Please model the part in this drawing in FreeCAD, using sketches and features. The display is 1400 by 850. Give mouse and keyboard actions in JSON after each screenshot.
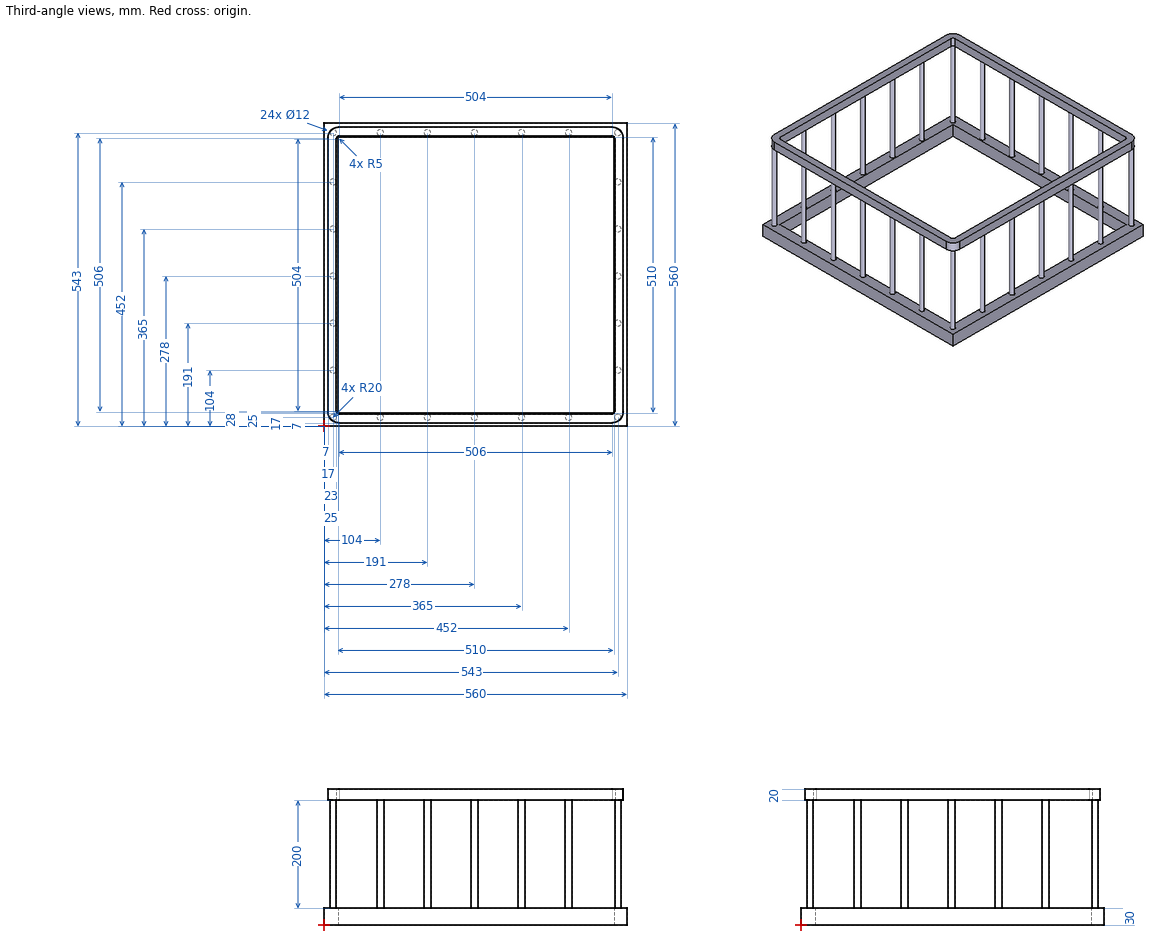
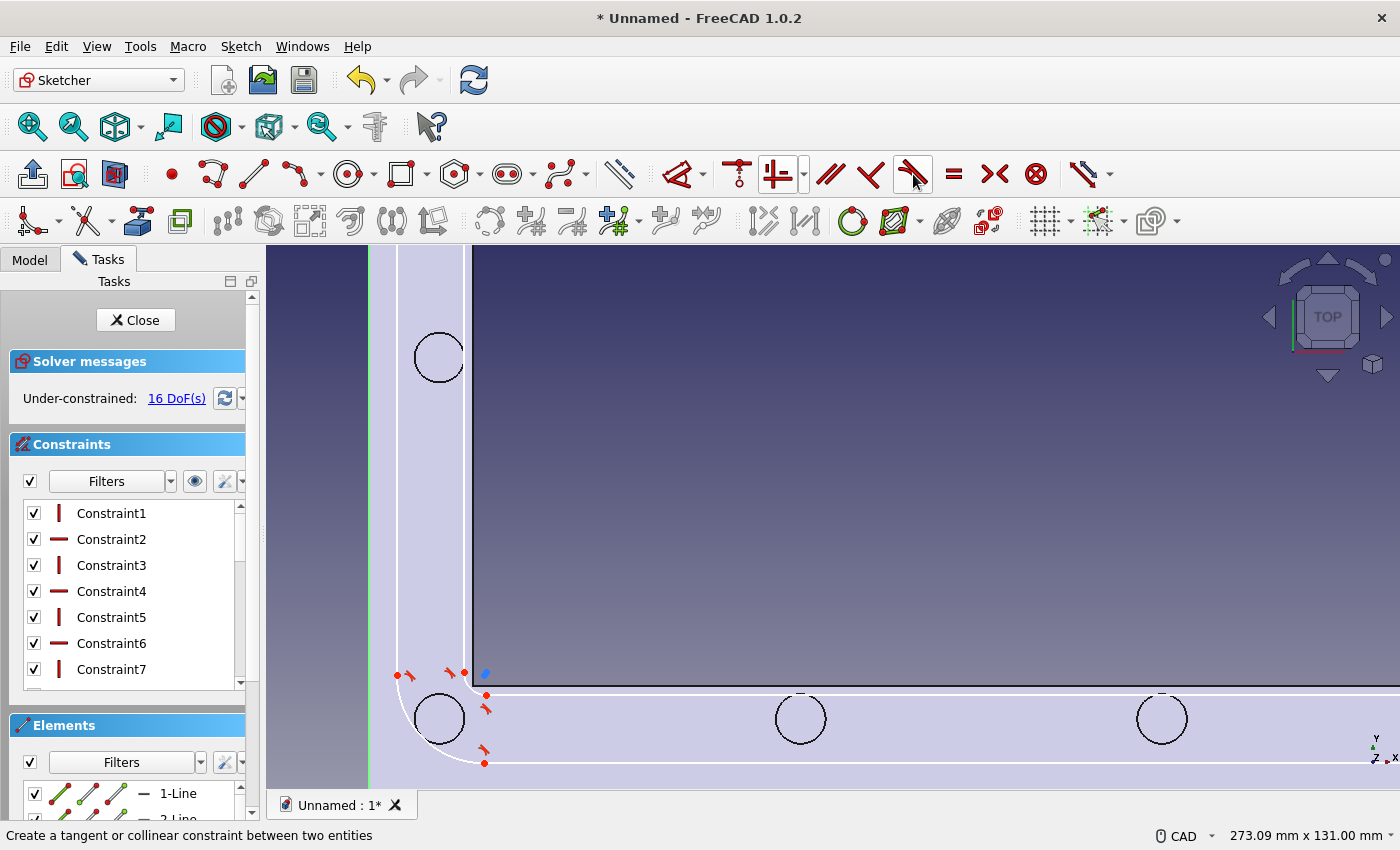
{"action": "left_click", "coordinate": [407, 715]}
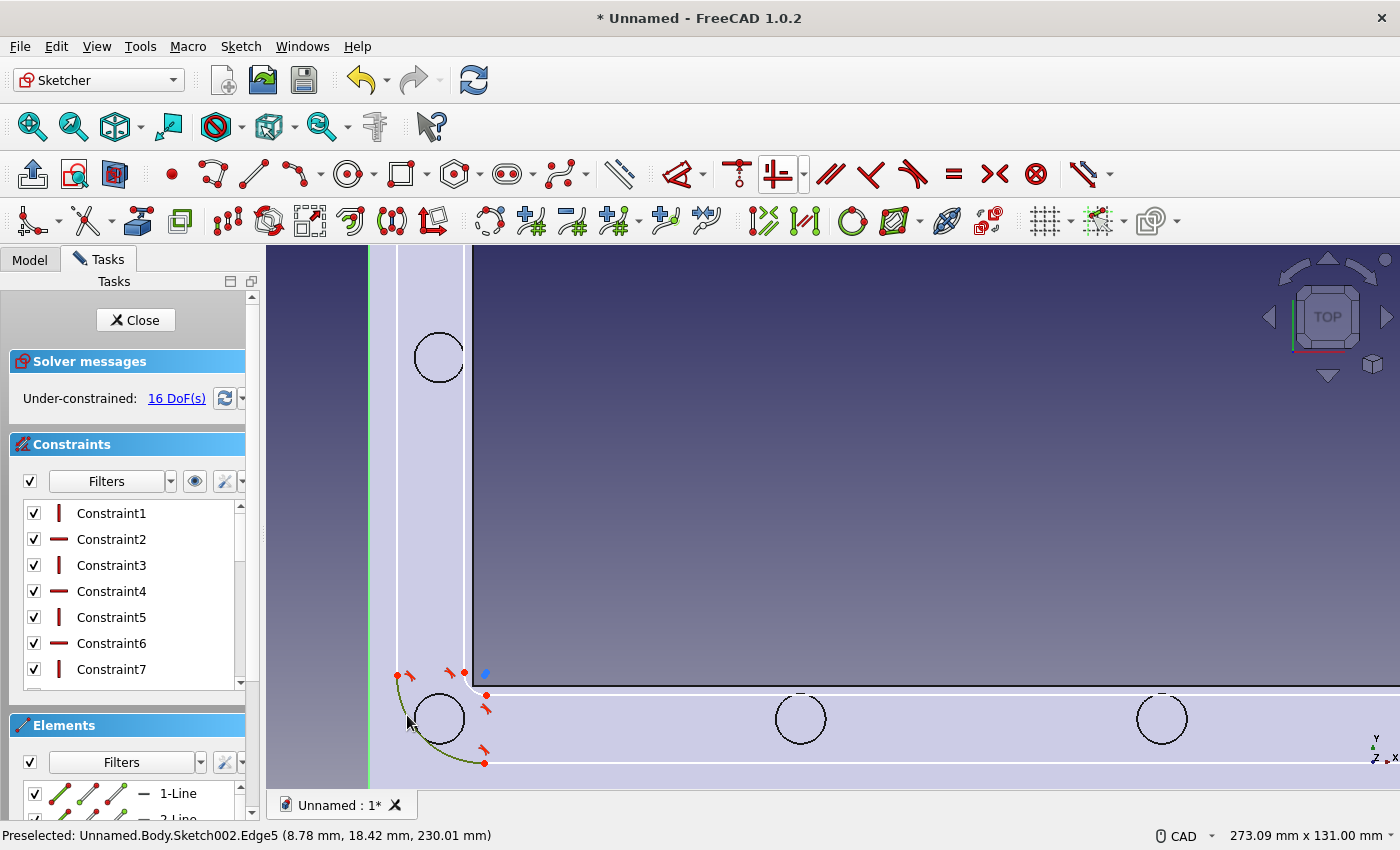
{"action": "scroll", "coordinate": [615, 690], "scroll_direction": "down", "scroll_amount": 9}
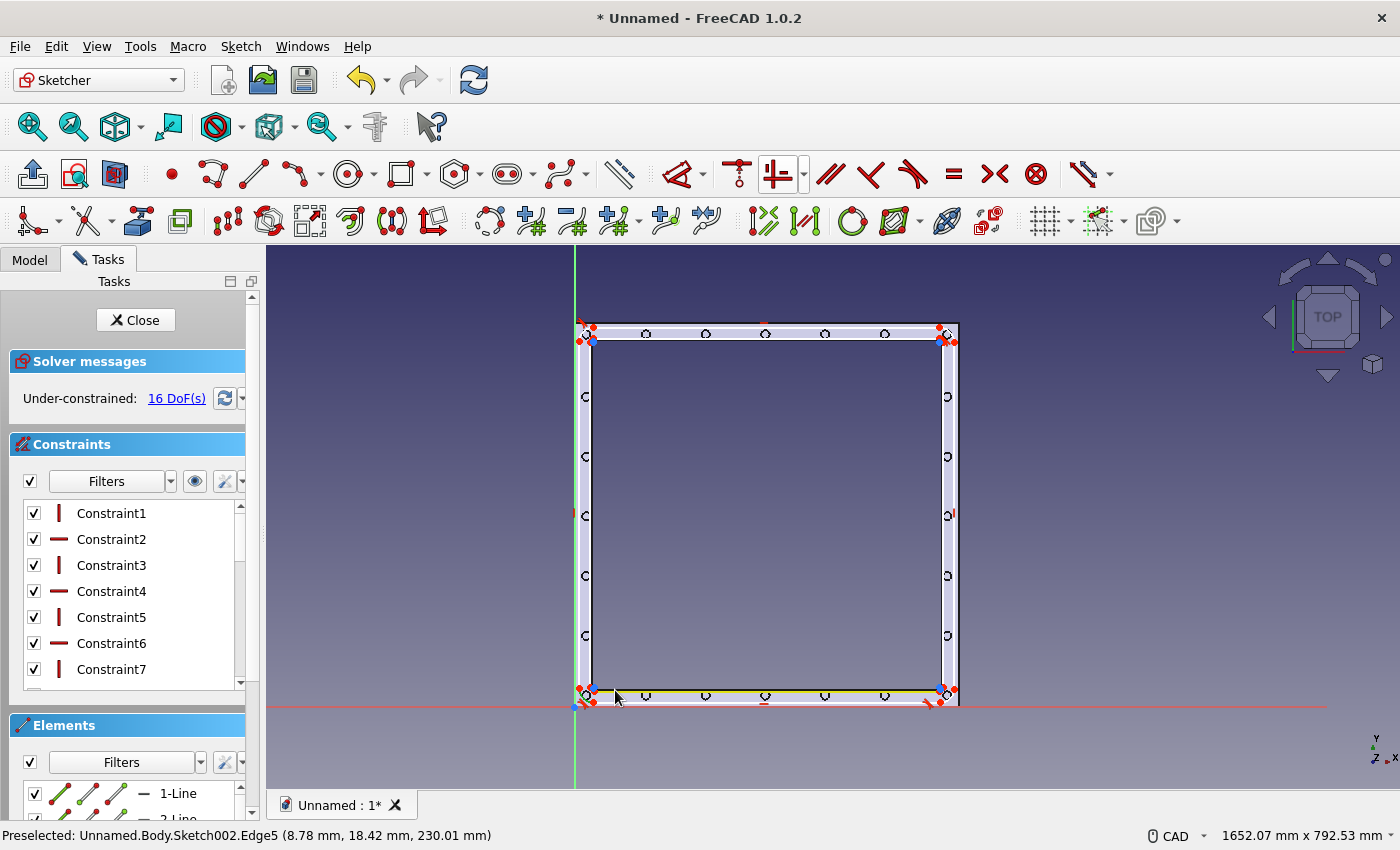
{"action": "scroll", "coordinate": [947, 701], "scroll_direction": "up", "scroll_amount": 5}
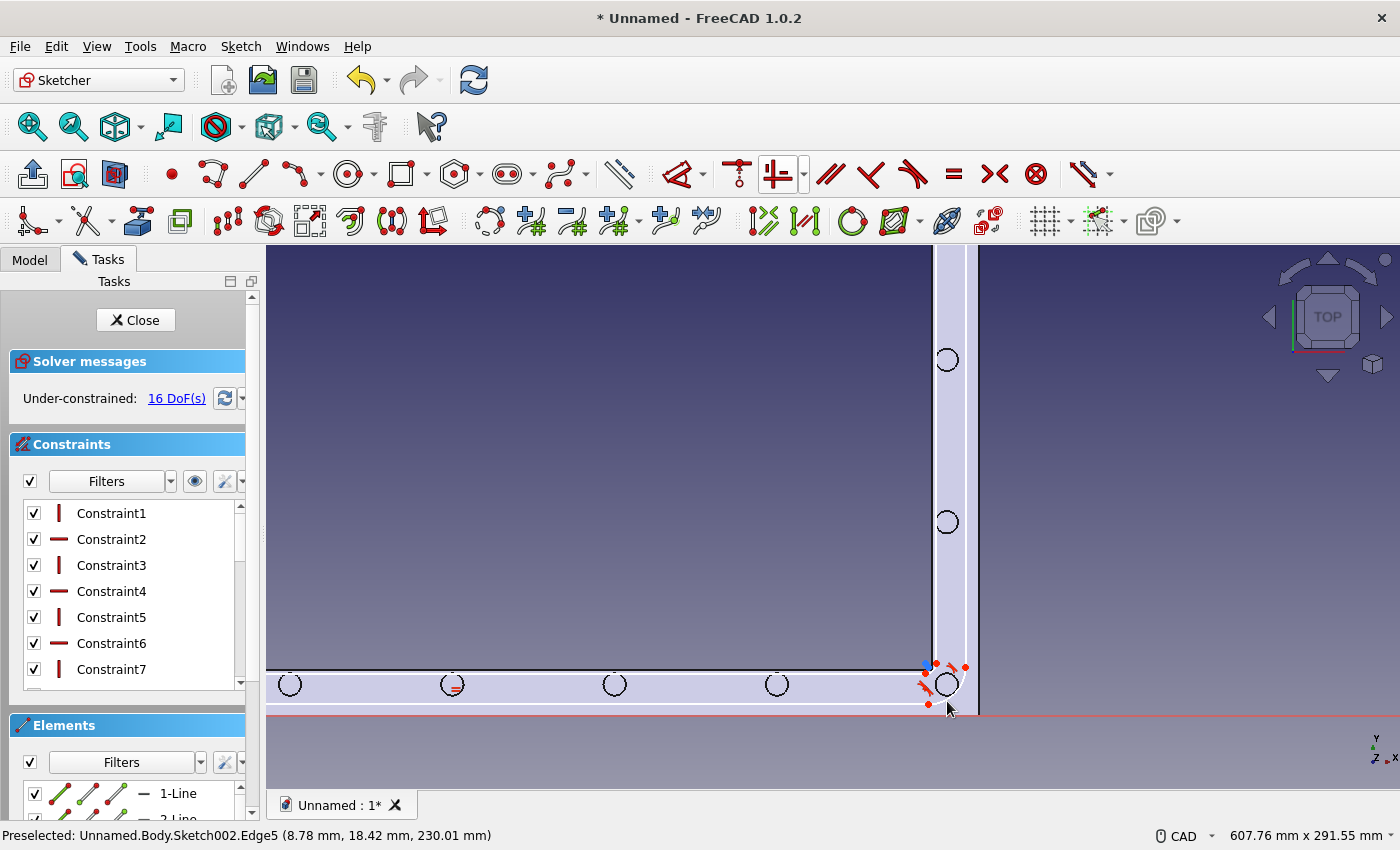
{"action": "left_click", "coordinate": [945, 700]}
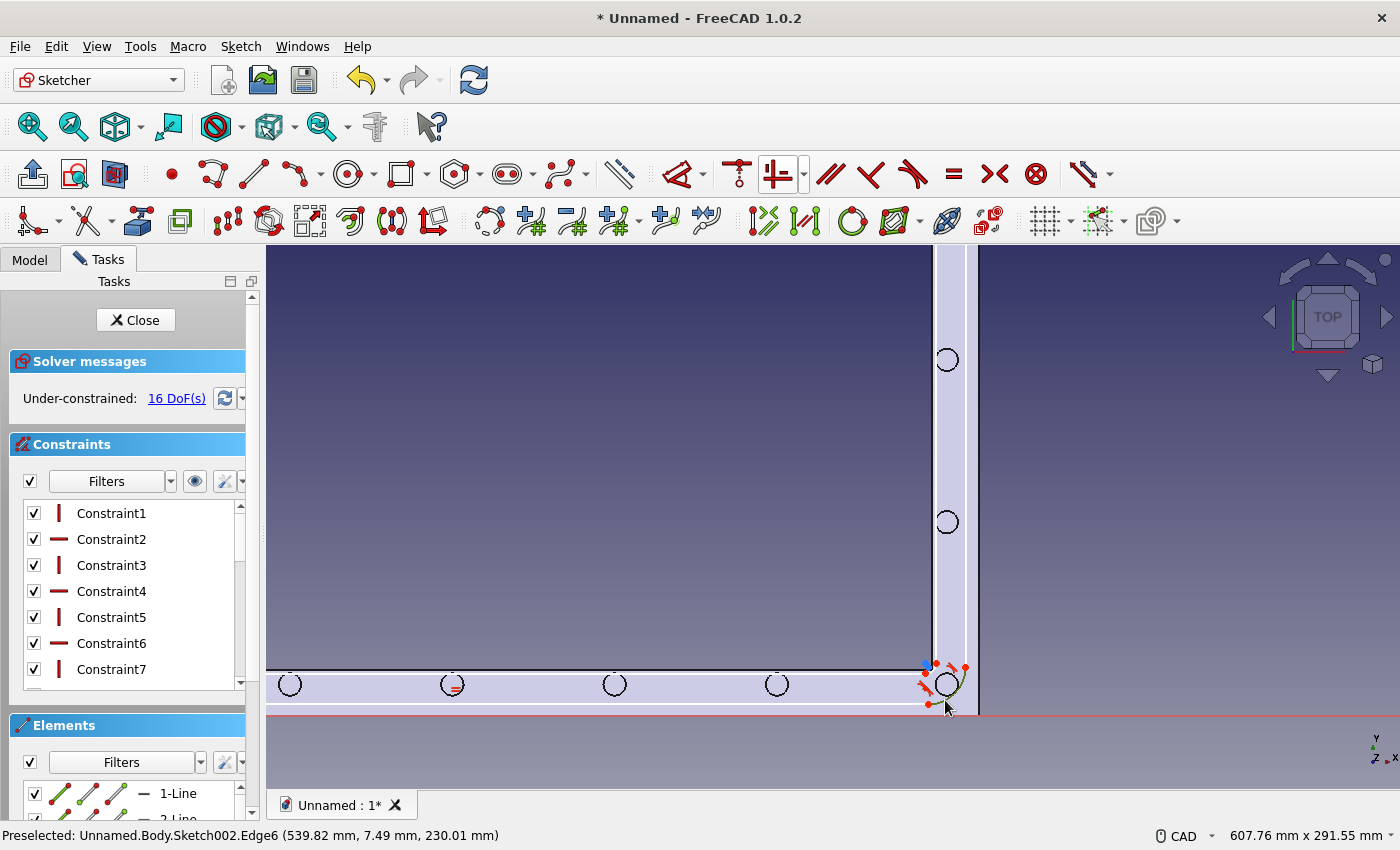
{"action": "scroll", "coordinate": [948, 701], "scroll_direction": "down", "scroll_amount": 5}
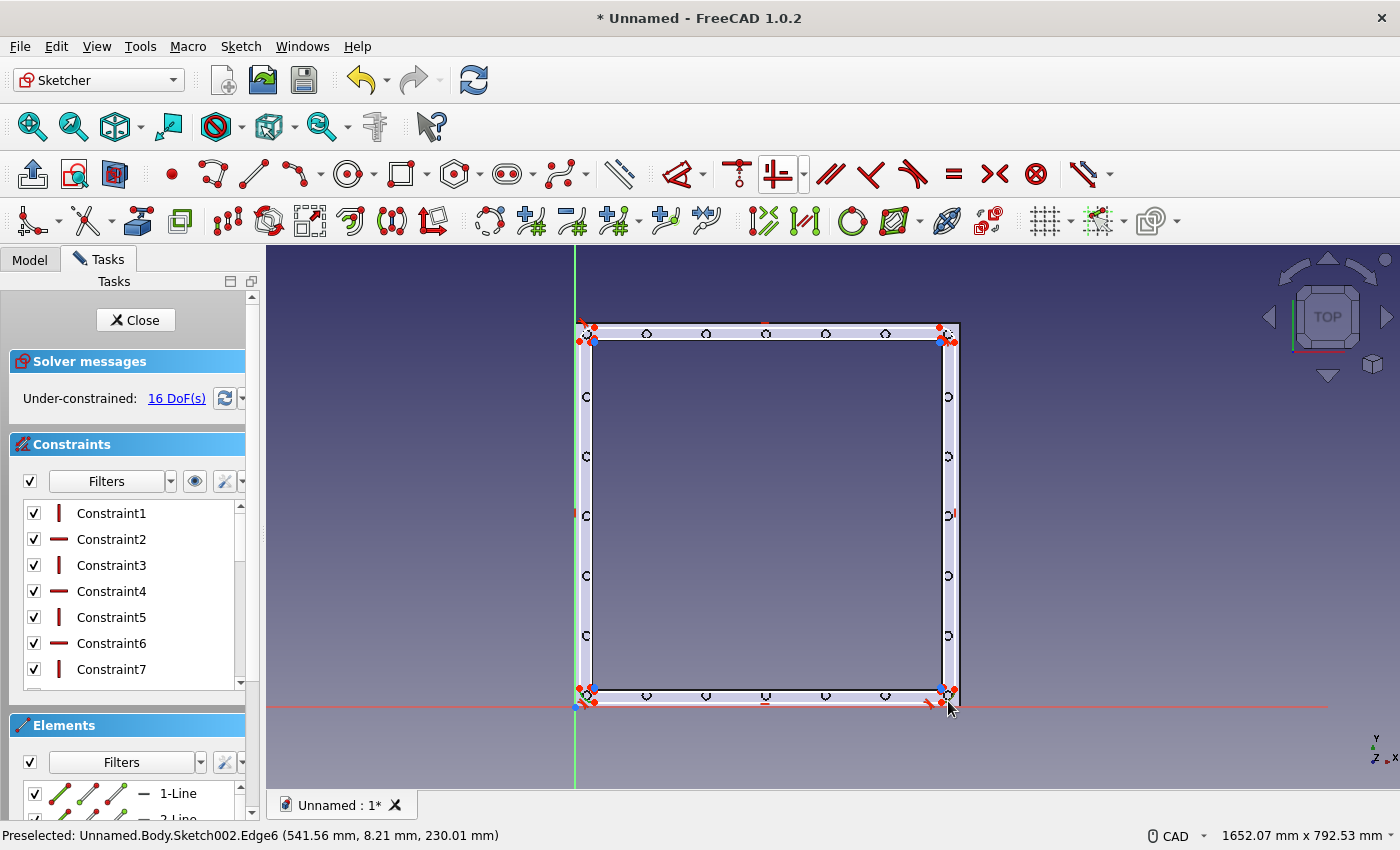
{"action": "scroll", "coordinate": [953, 336], "scroll_direction": "up", "scroll_amount": 4}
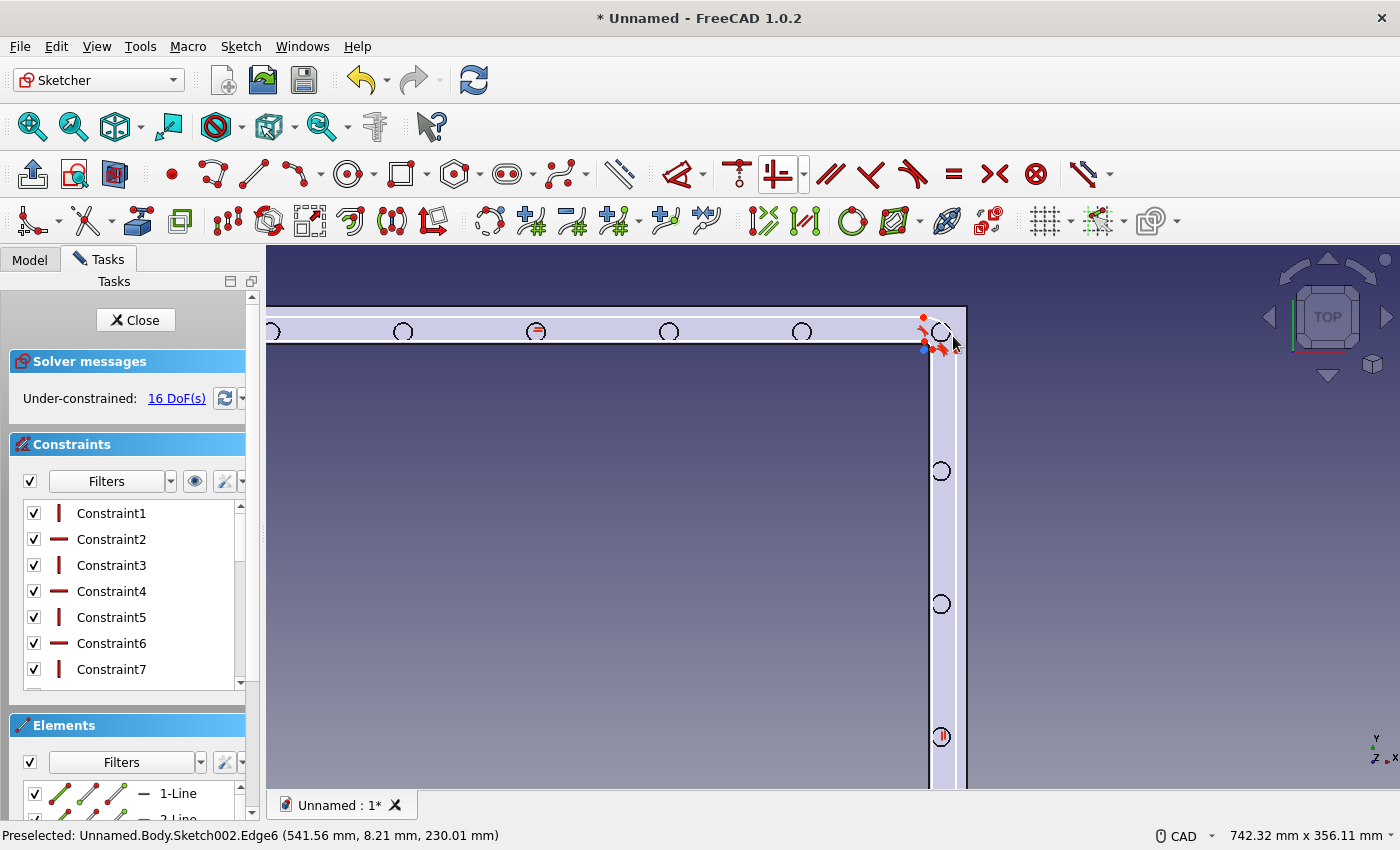
{"action": "left_click", "coordinate": [953, 335]}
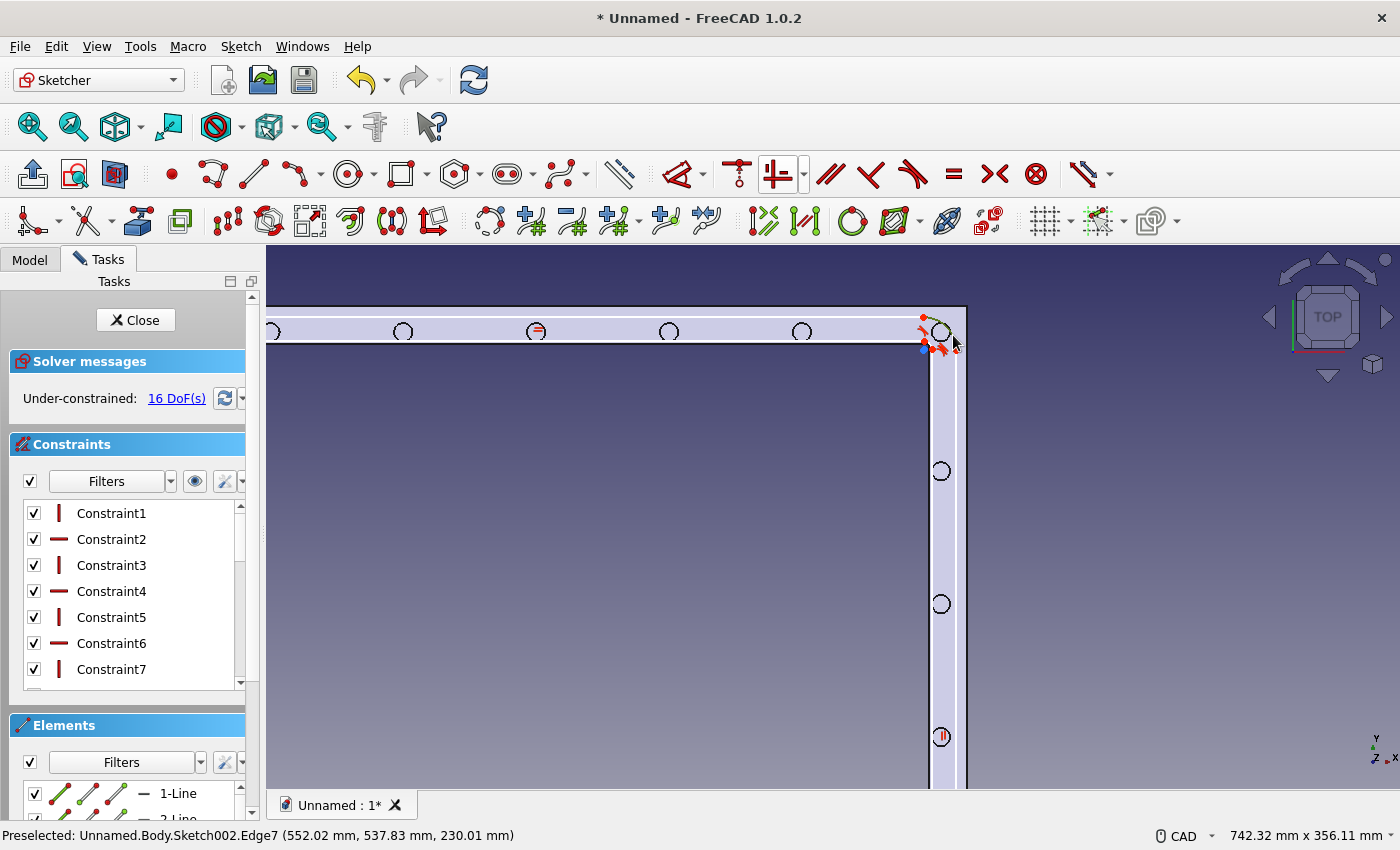
{"action": "scroll", "coordinate": [953, 336], "scroll_direction": "down", "scroll_amount": 4}